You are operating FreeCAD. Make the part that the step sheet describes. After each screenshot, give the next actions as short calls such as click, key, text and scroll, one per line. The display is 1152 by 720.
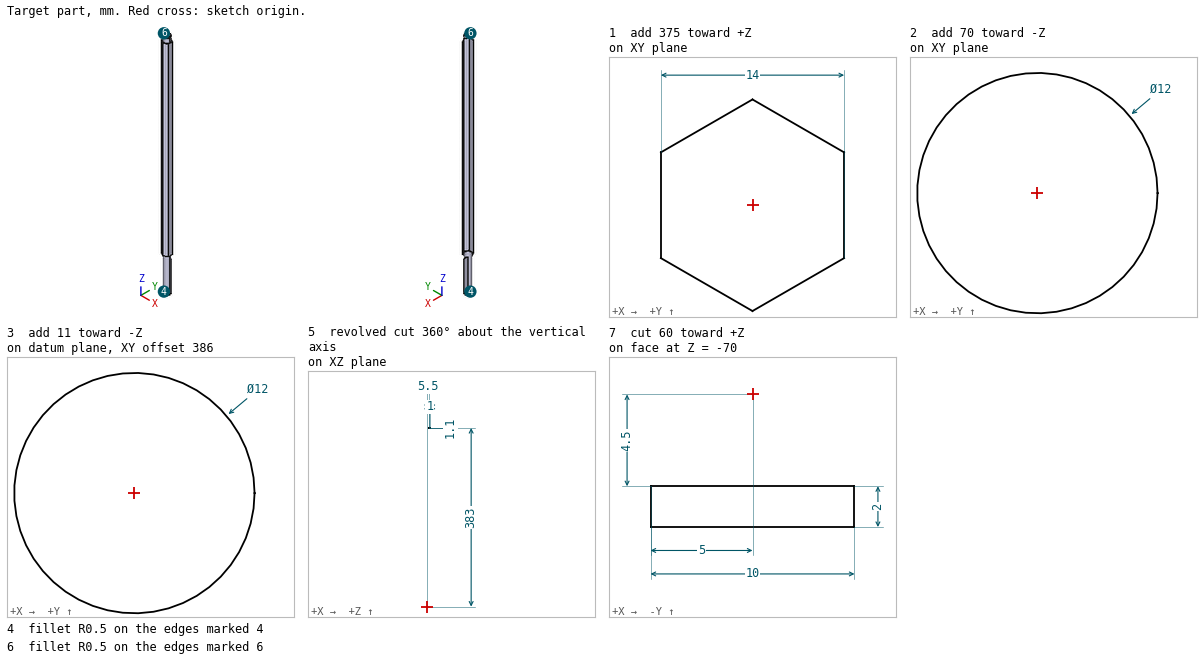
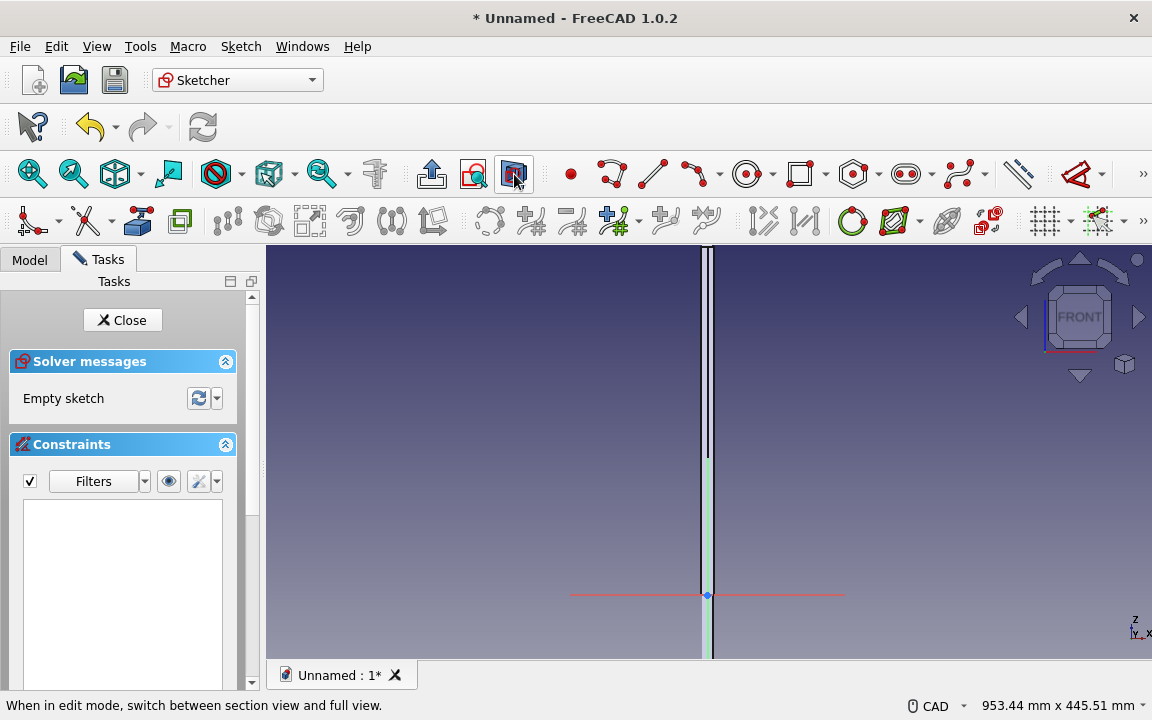
scroll(640, 452, down, 5)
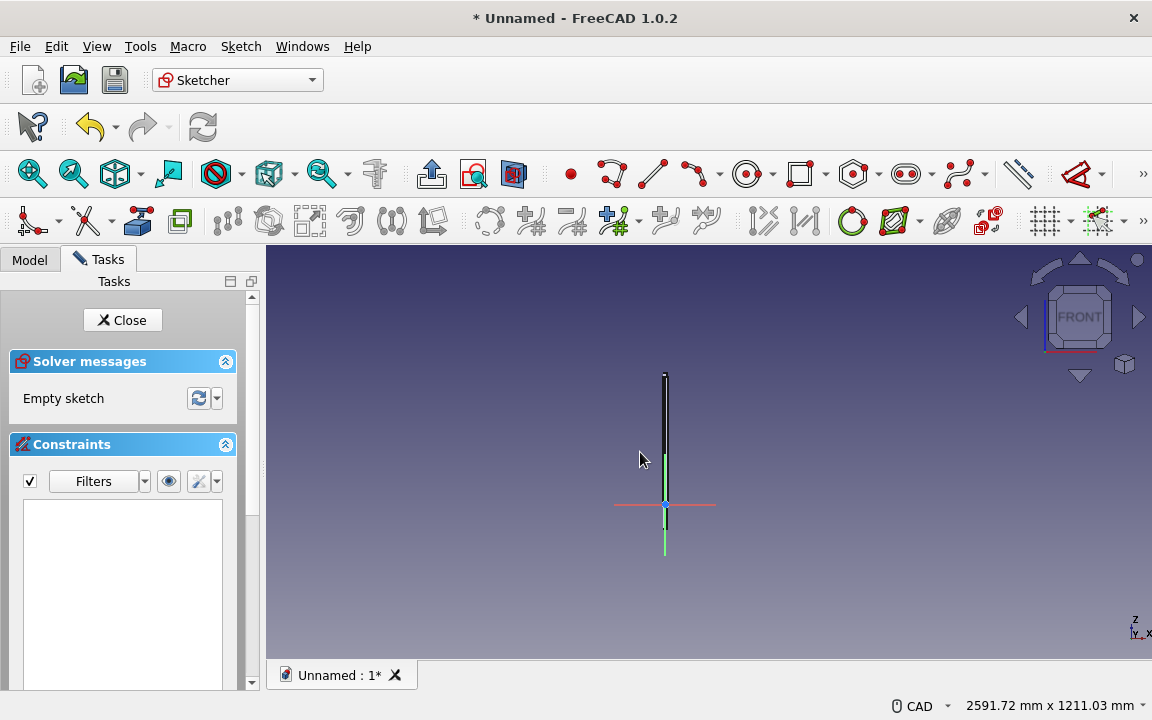
scroll(669, 370, up, 15)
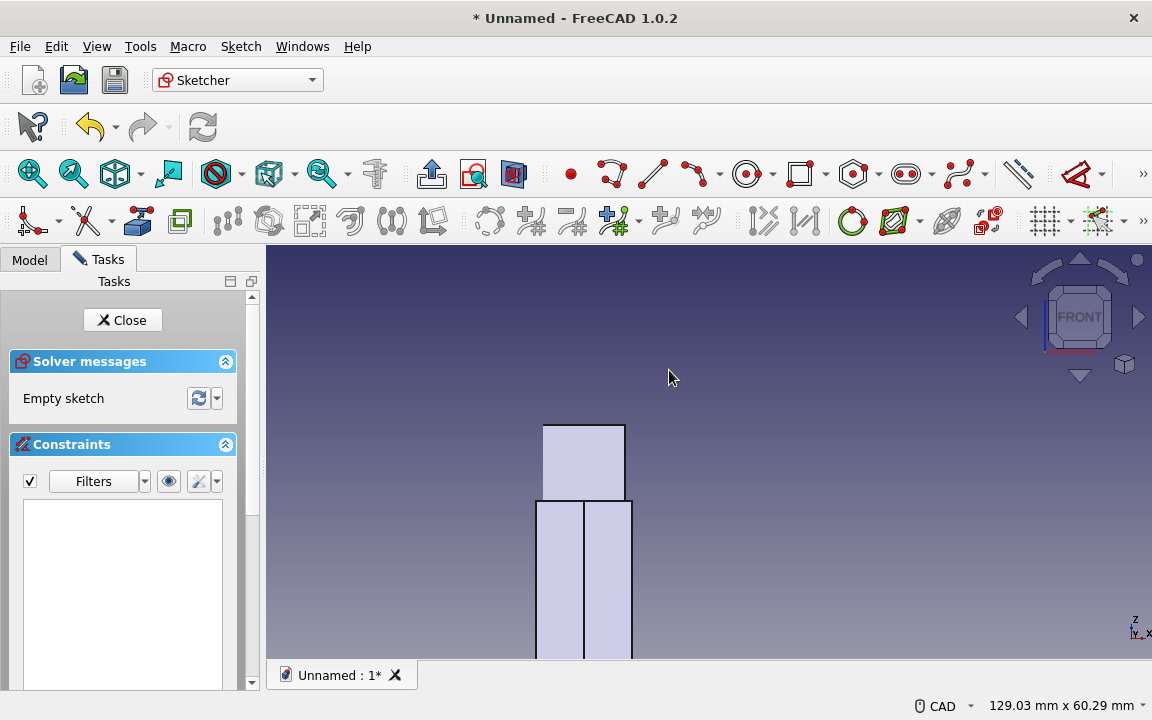
scroll(624, 441, up, 15)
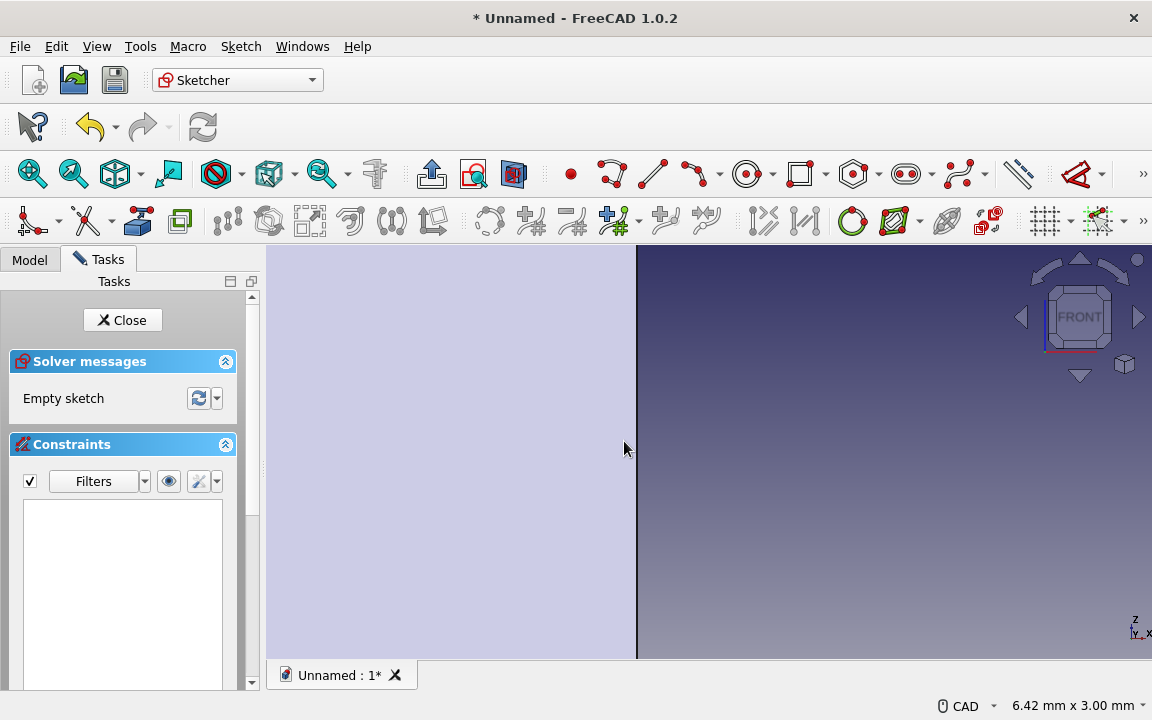
scroll(632, 449, up, 3)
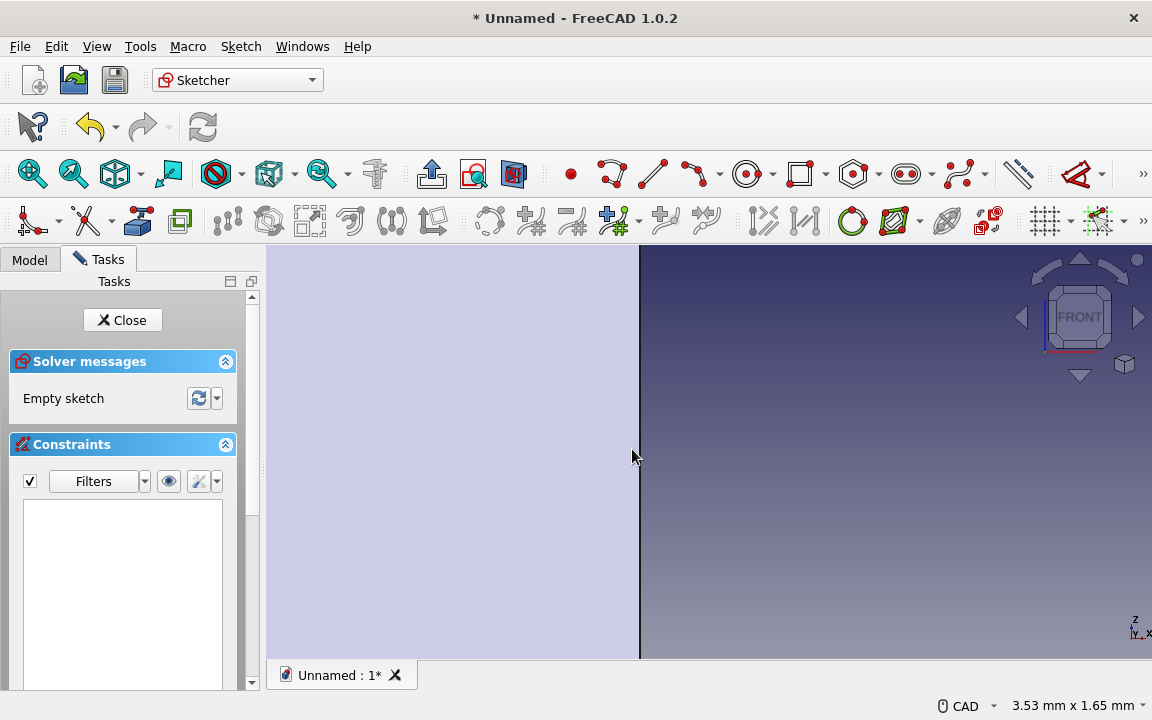
click(800, 174)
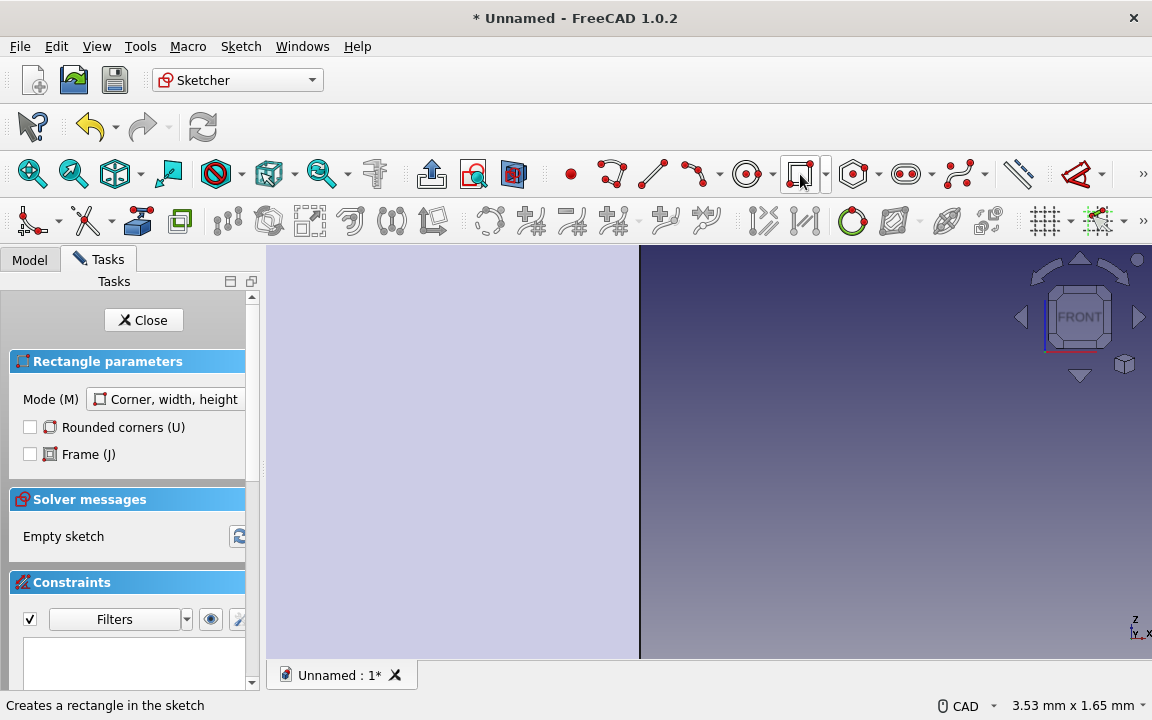
click(514, 314)
move(766, 590)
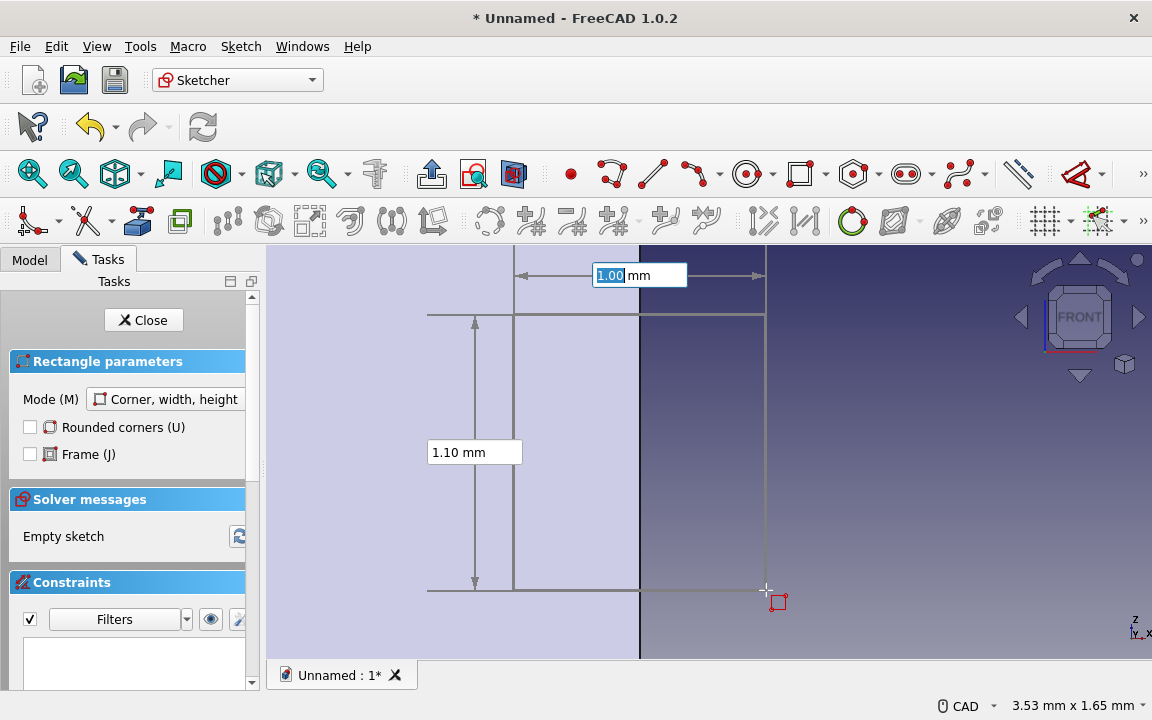
text(1)
key(Tab)
text(1.1)
key(Return)
key(Escape)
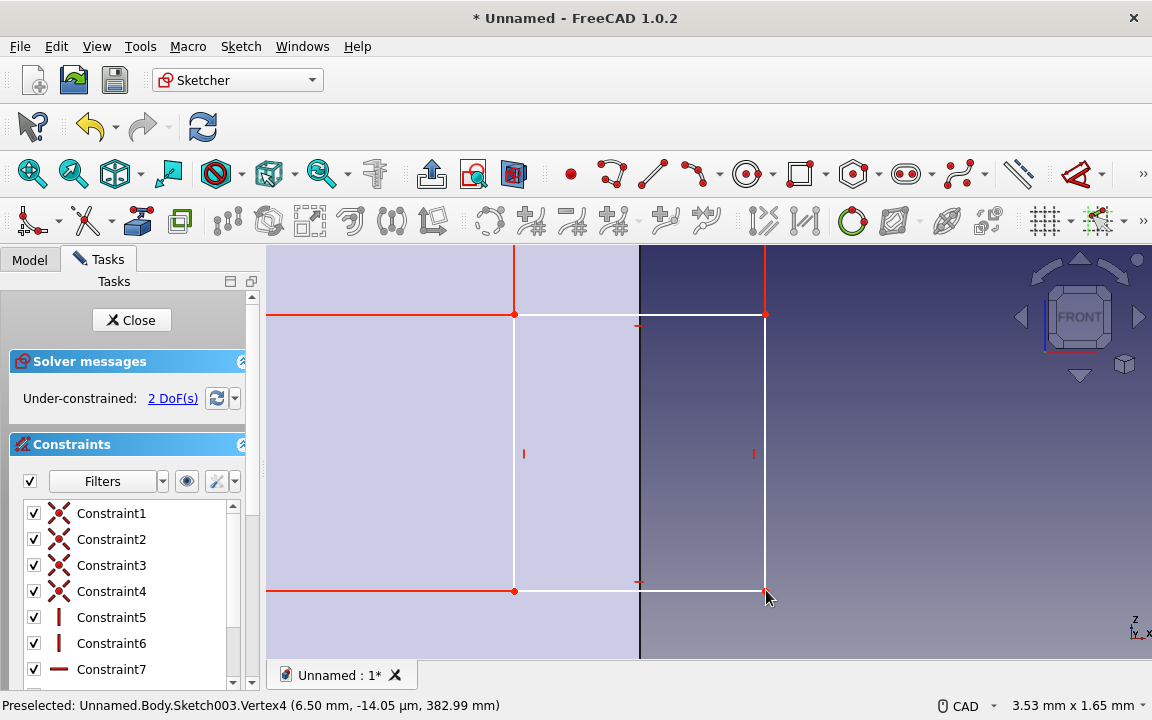
click(1076, 174)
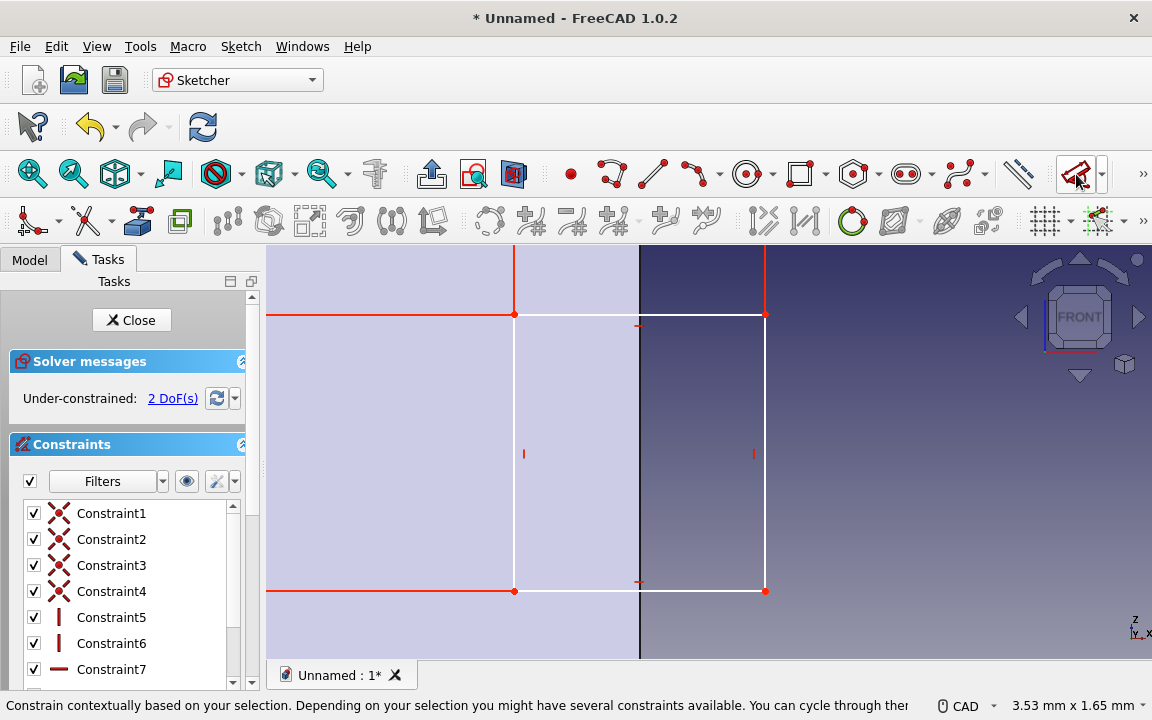
click(514, 315)
click(404, 281)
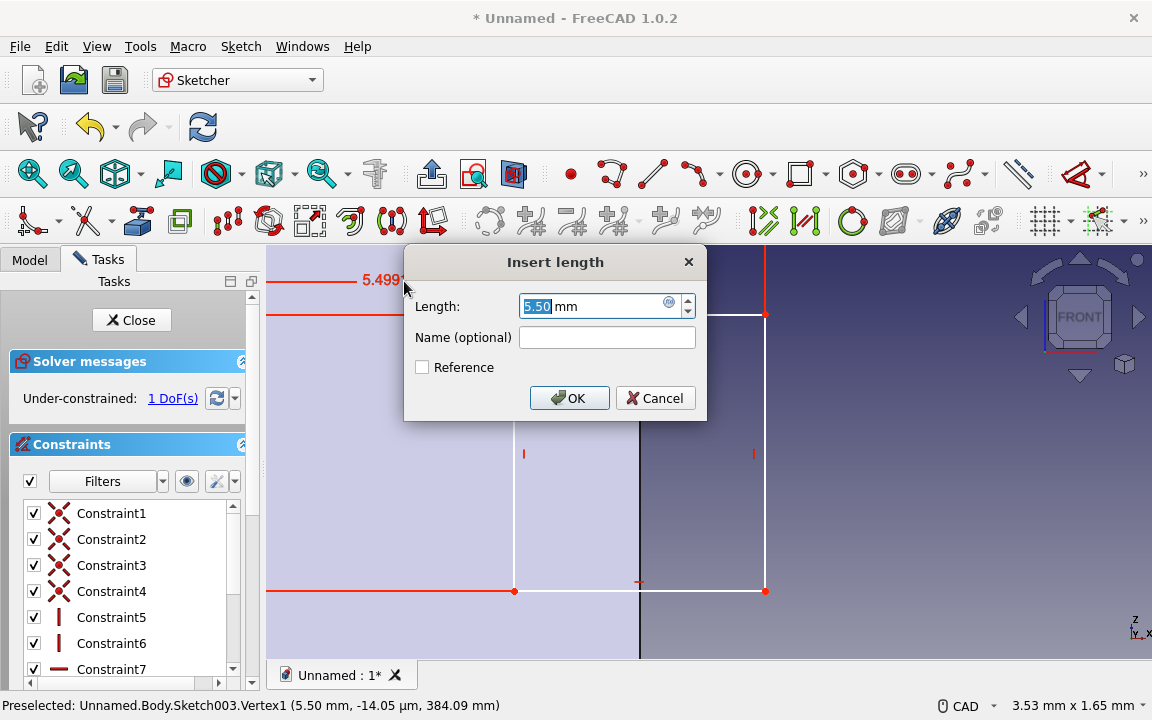
text(5.5)
key(Return)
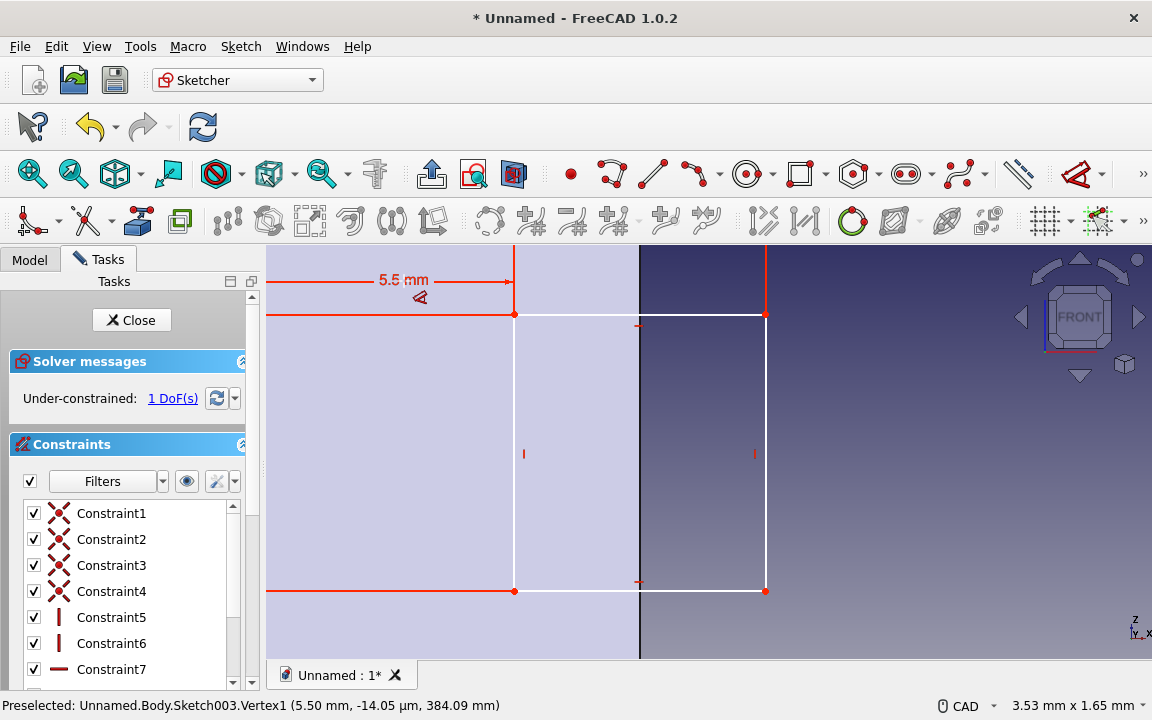
click(514, 591)
click(548, 611)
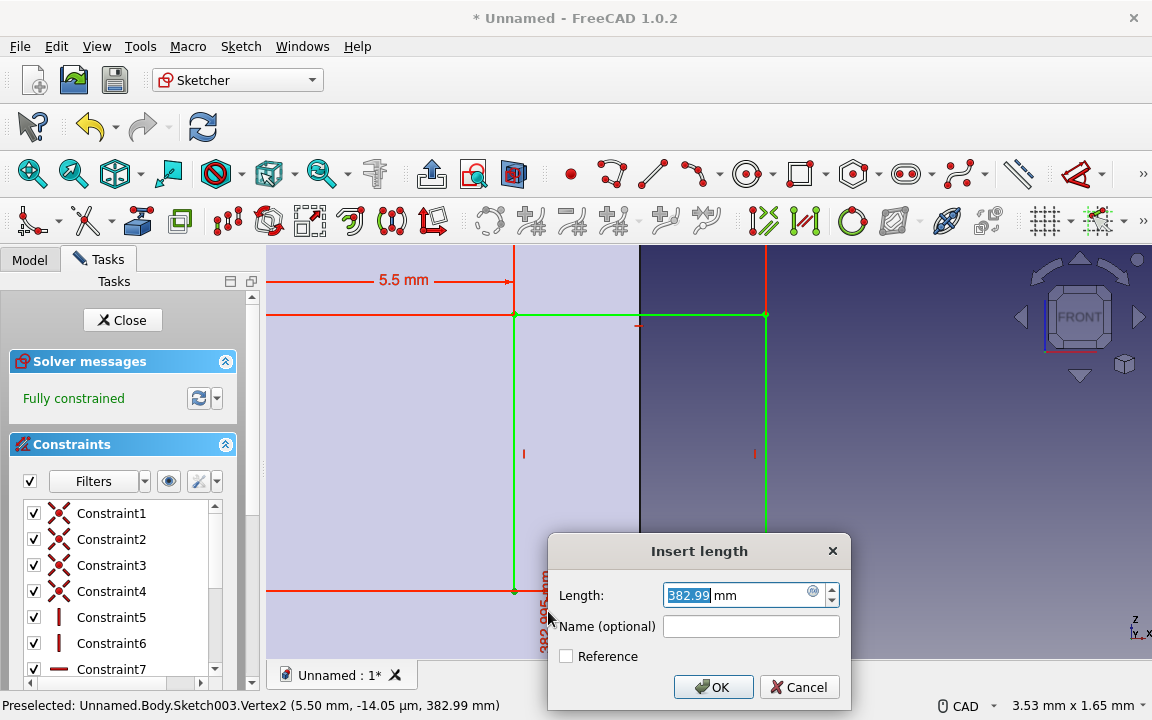
text(383)
key(Return)
key(Escape)